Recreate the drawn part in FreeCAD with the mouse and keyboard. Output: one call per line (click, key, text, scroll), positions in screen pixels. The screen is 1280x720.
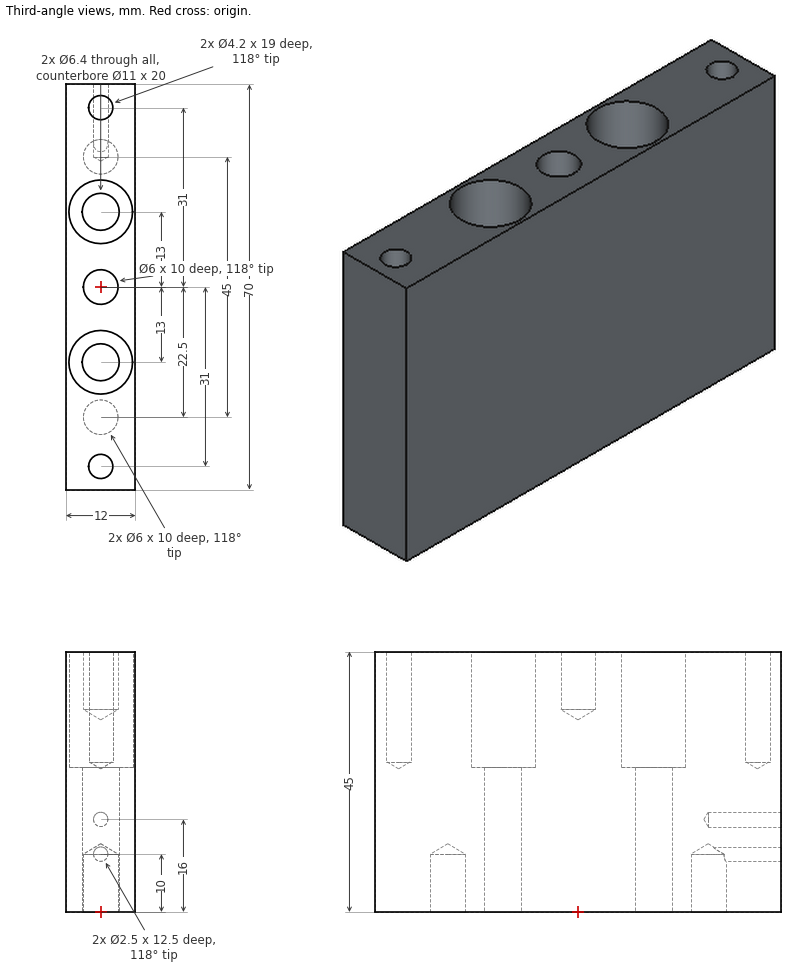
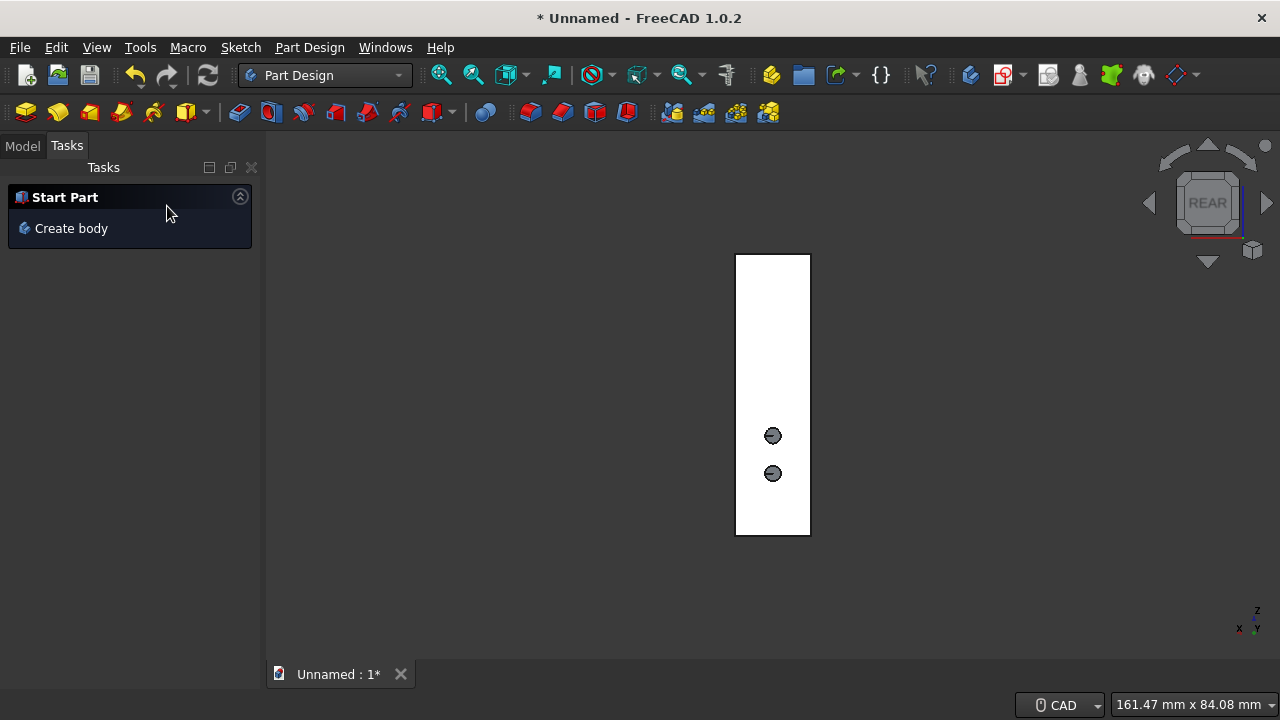
key(0)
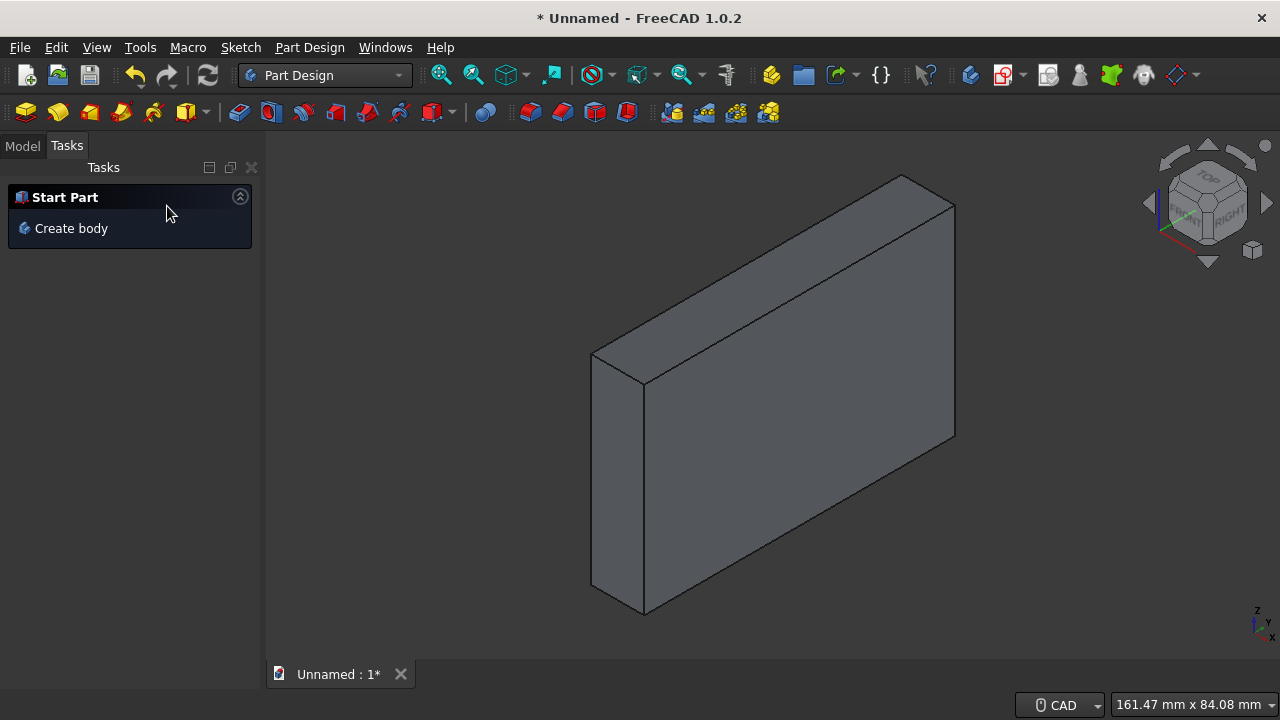
click(862, 227)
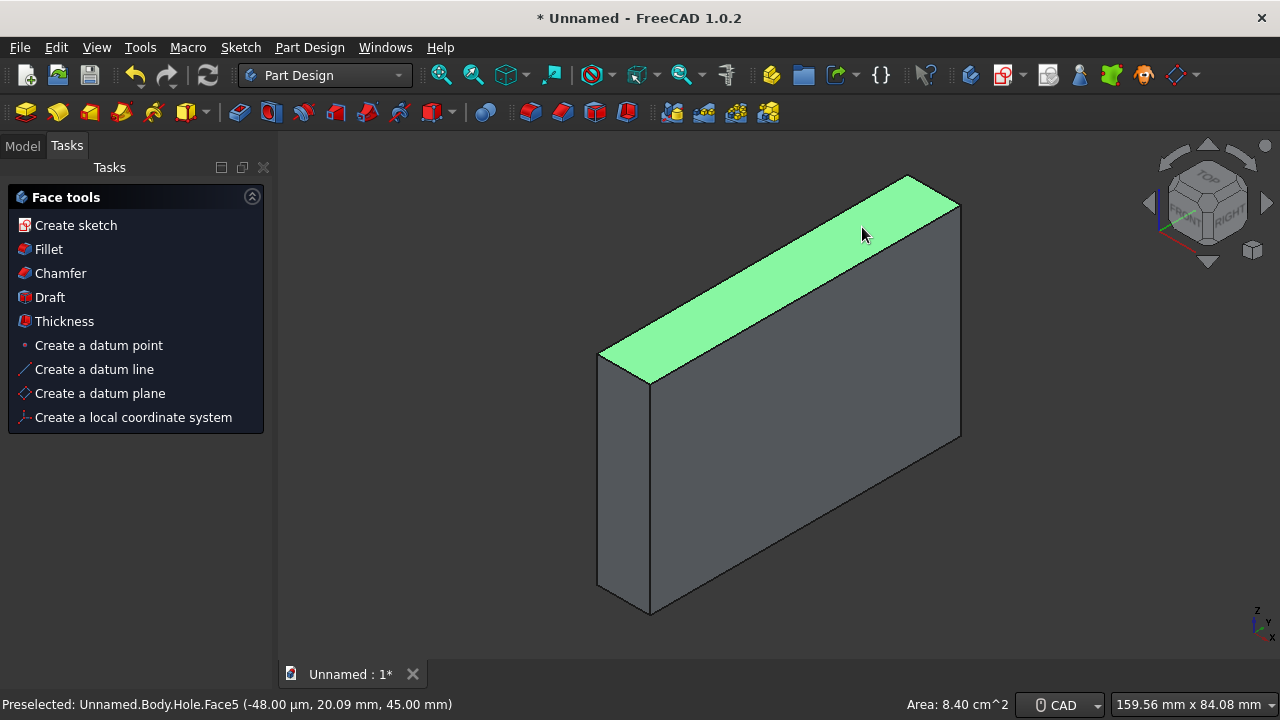
click(1004, 76)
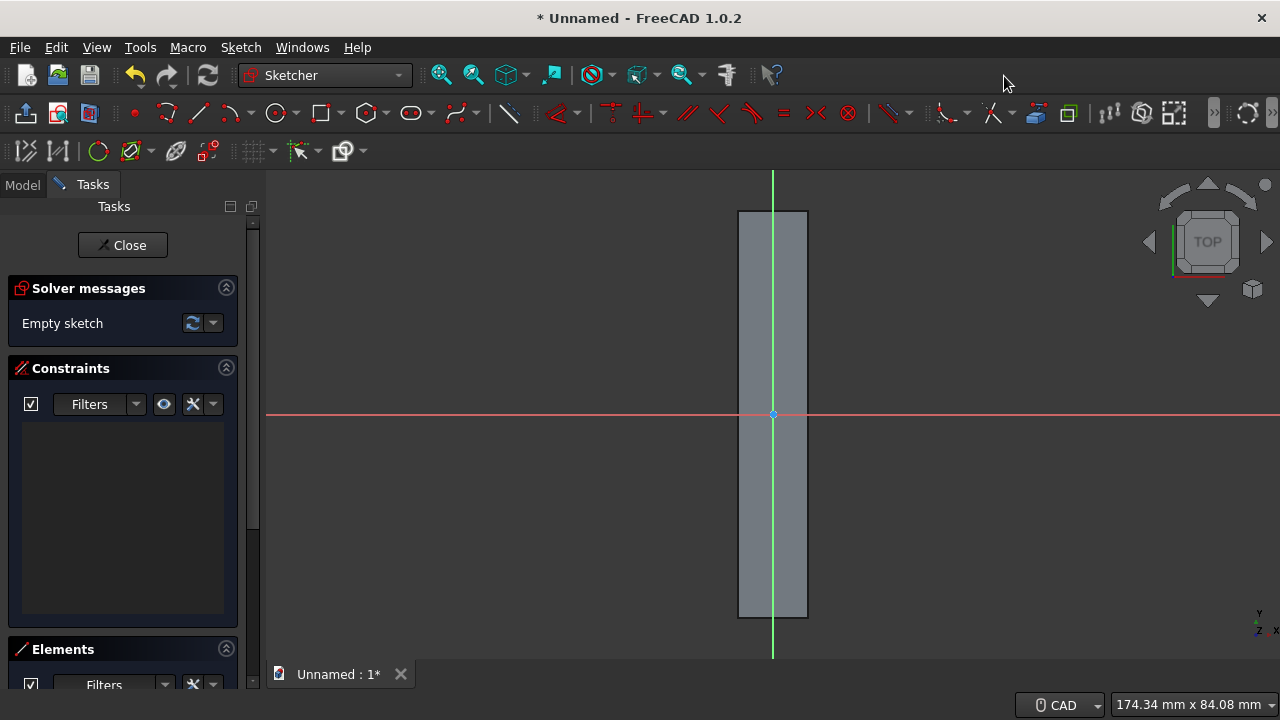
scroll(395, 415, down, 1)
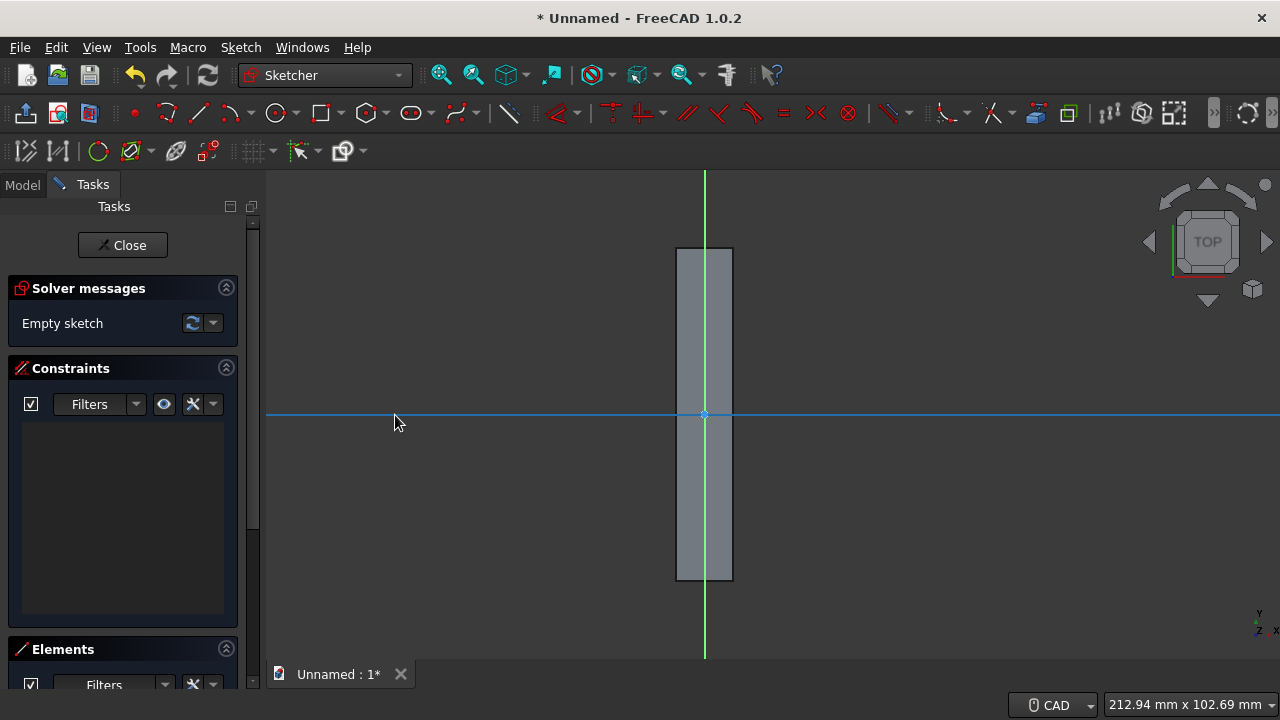
click(276, 114)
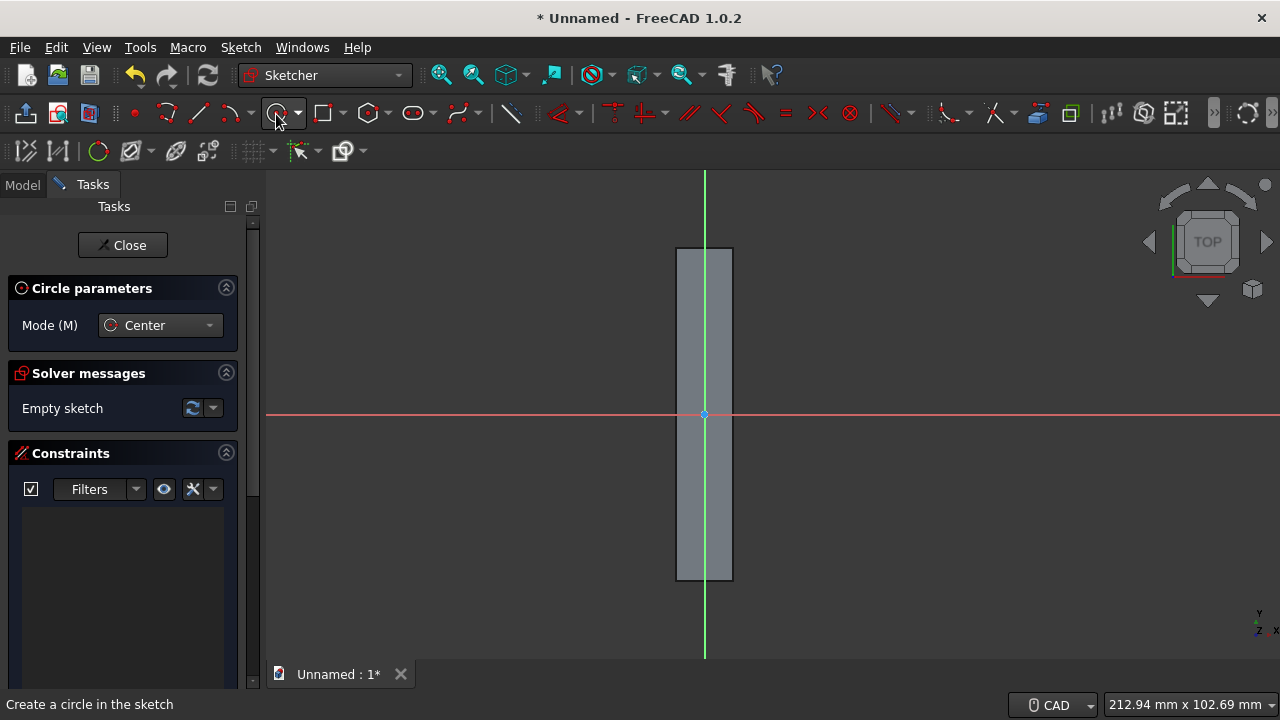
scroll(705, 267, up, 5)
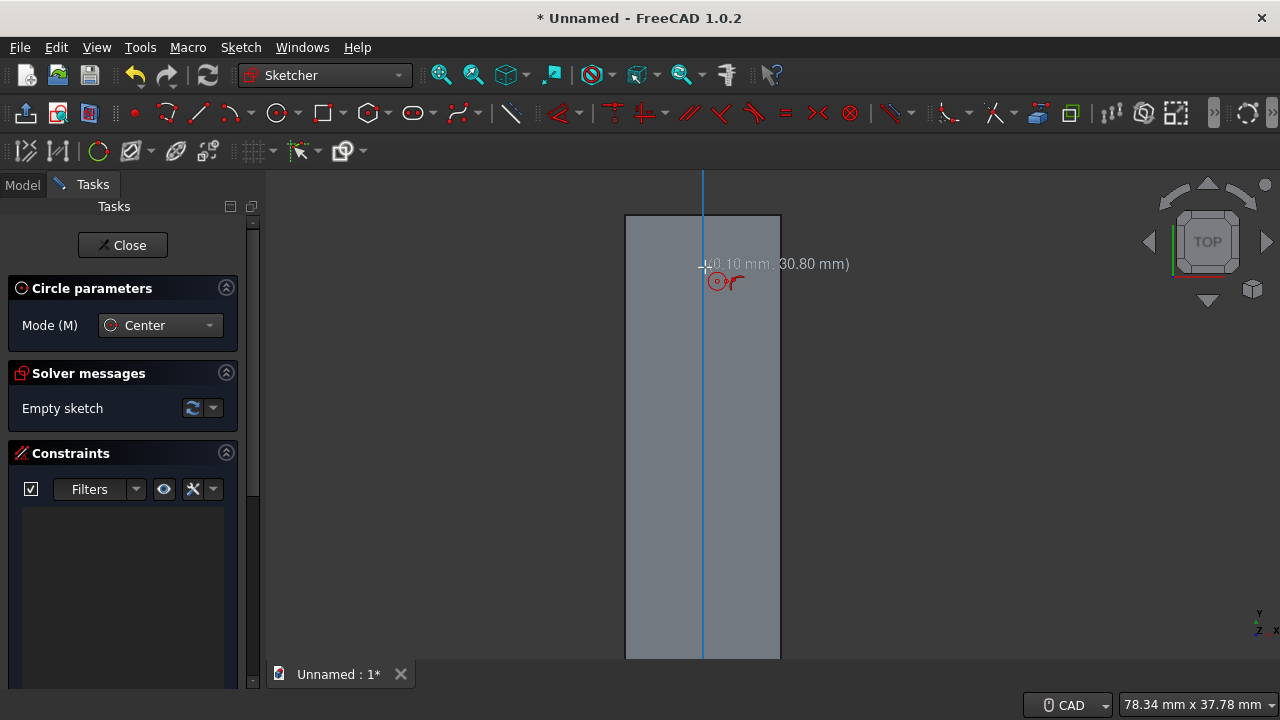
click(703, 267)
move(722, 248)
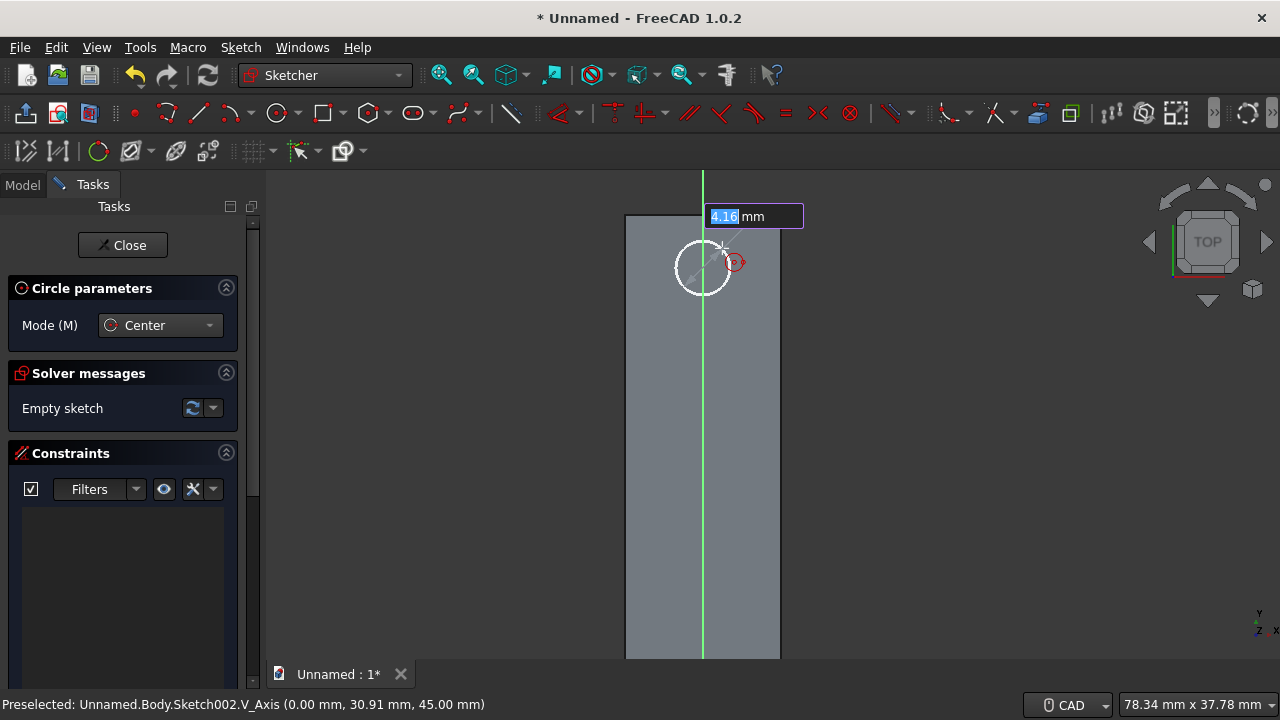
text(4.2)
key(Return)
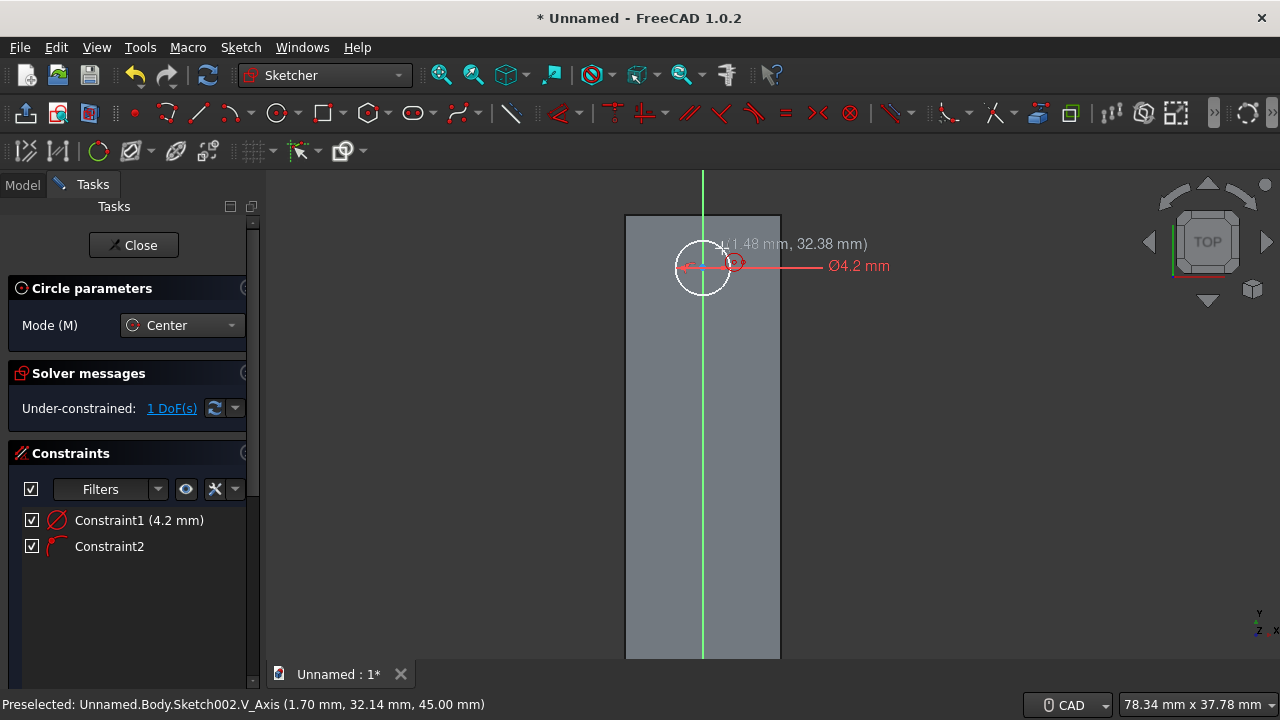
scroll(705, 267, down, 5)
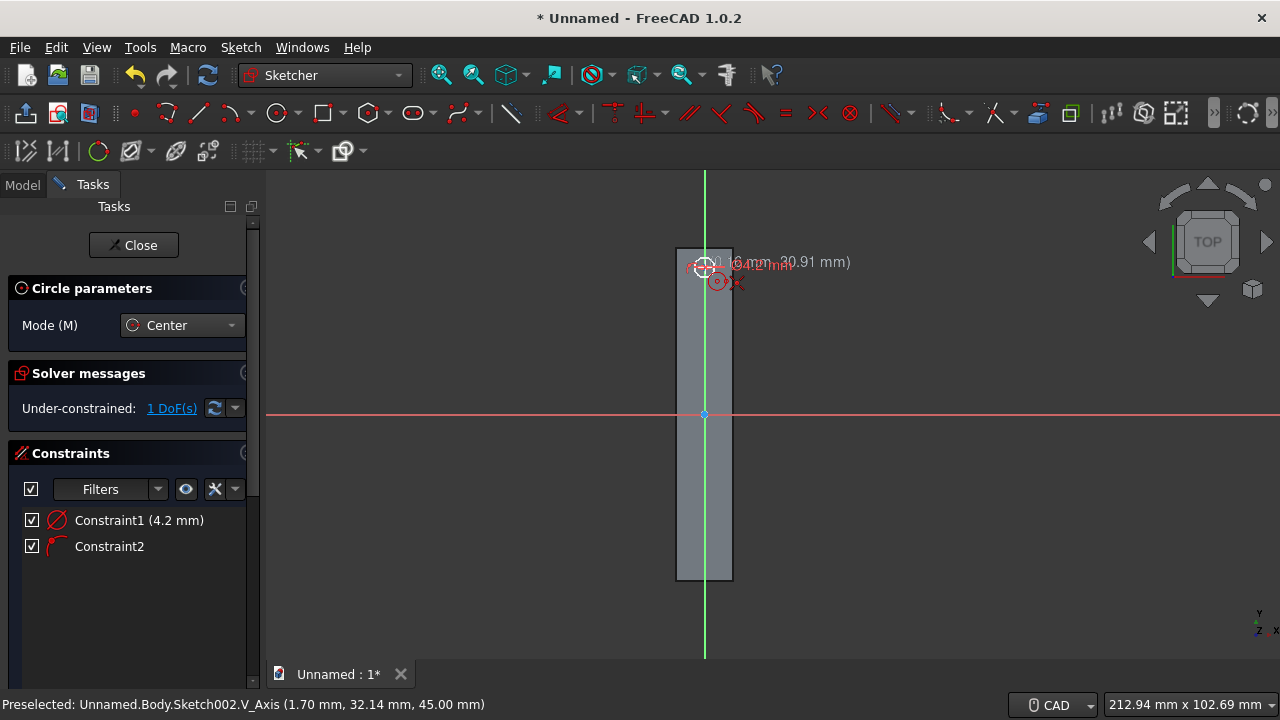
scroll(705, 562, up, 5)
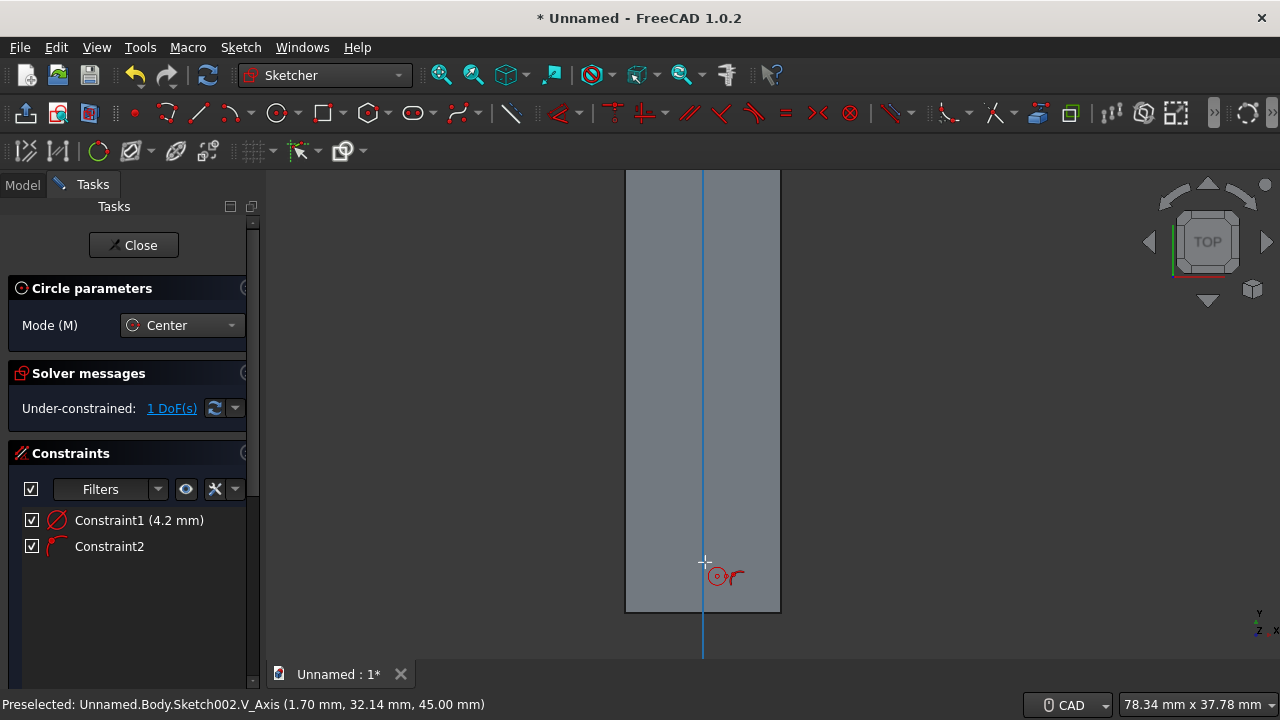
click(703, 561)
move(722, 542)